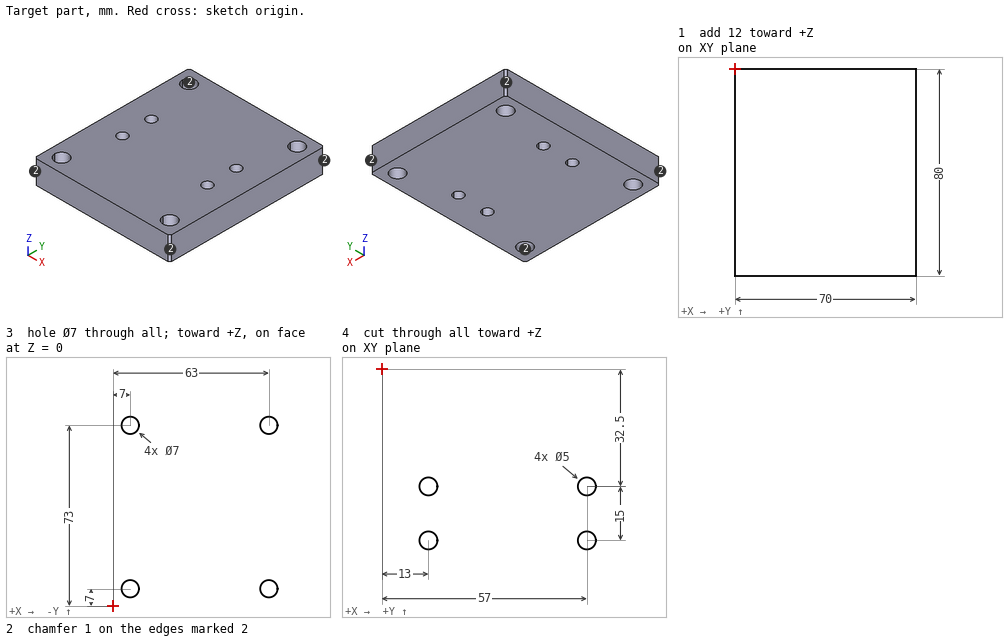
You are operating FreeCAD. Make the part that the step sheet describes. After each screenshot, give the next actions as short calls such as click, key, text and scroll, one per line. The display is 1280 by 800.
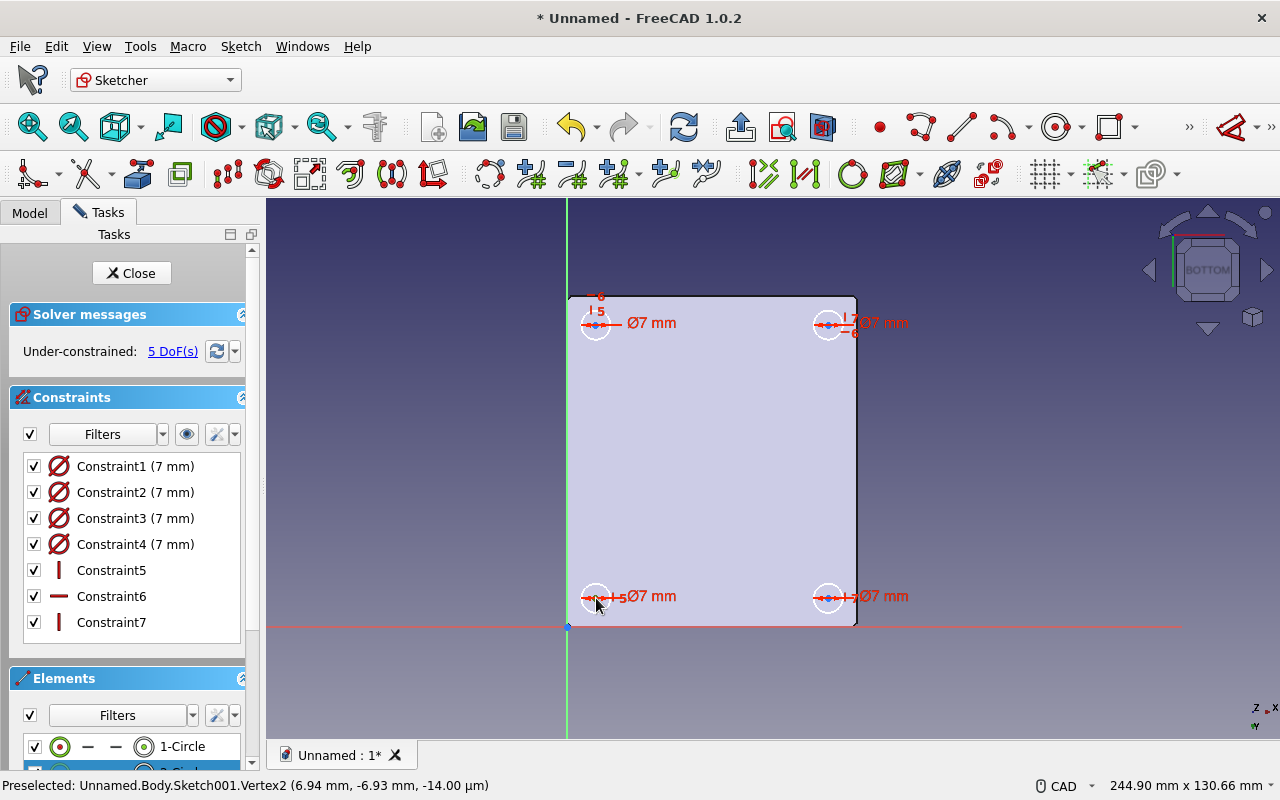
click(828, 598)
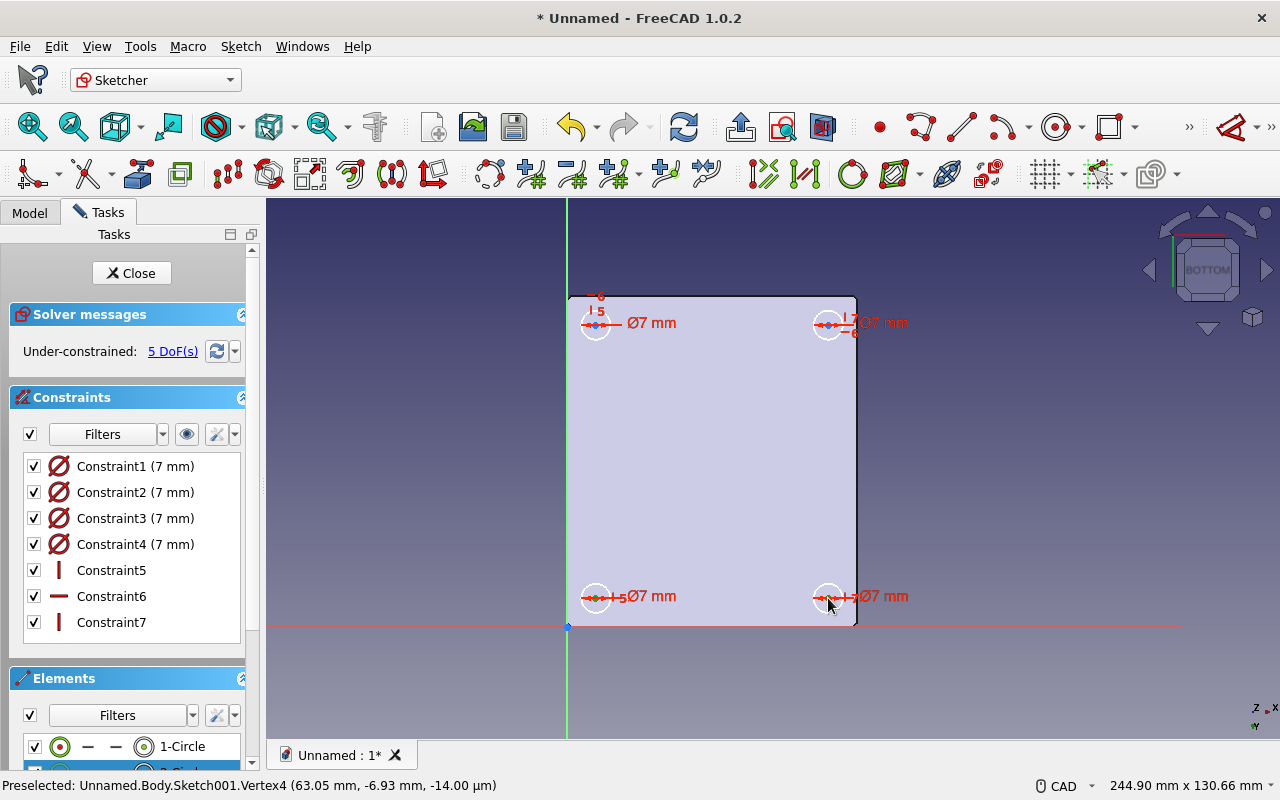
key(h)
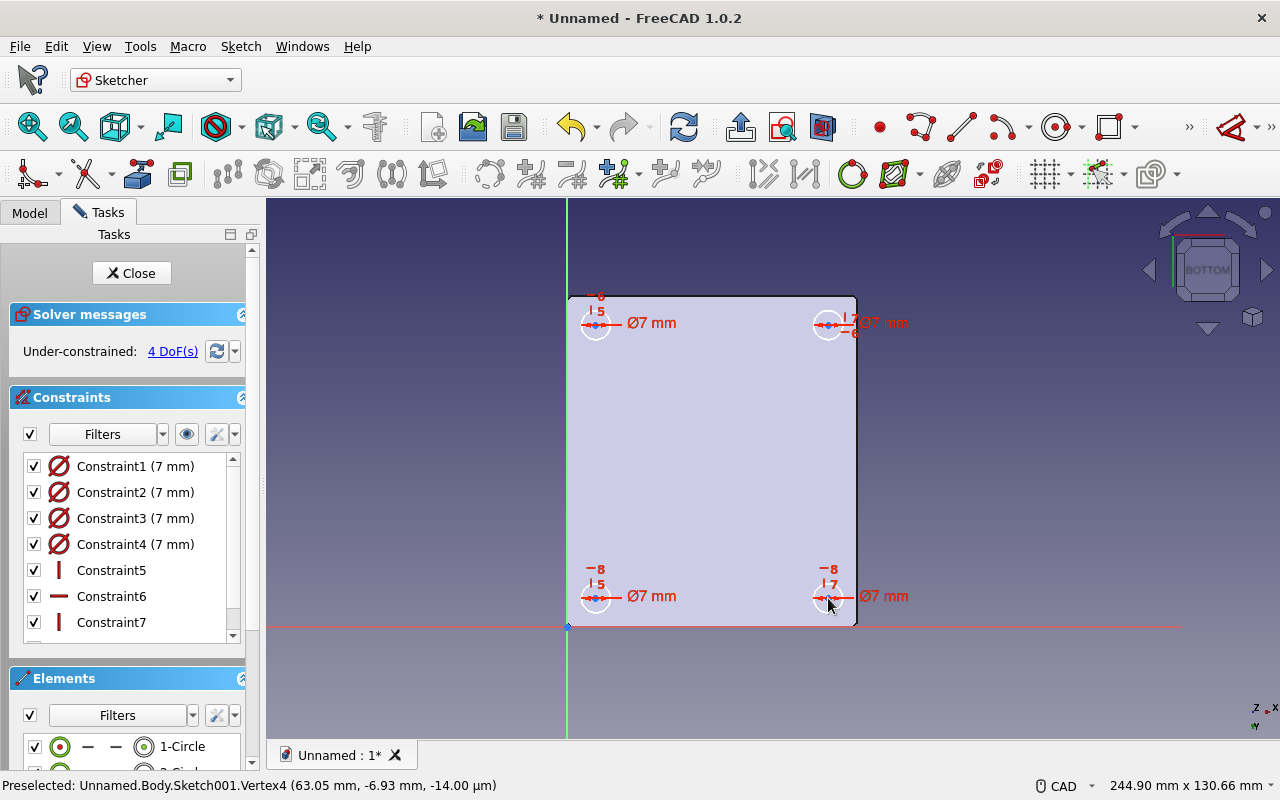
click(1230, 128)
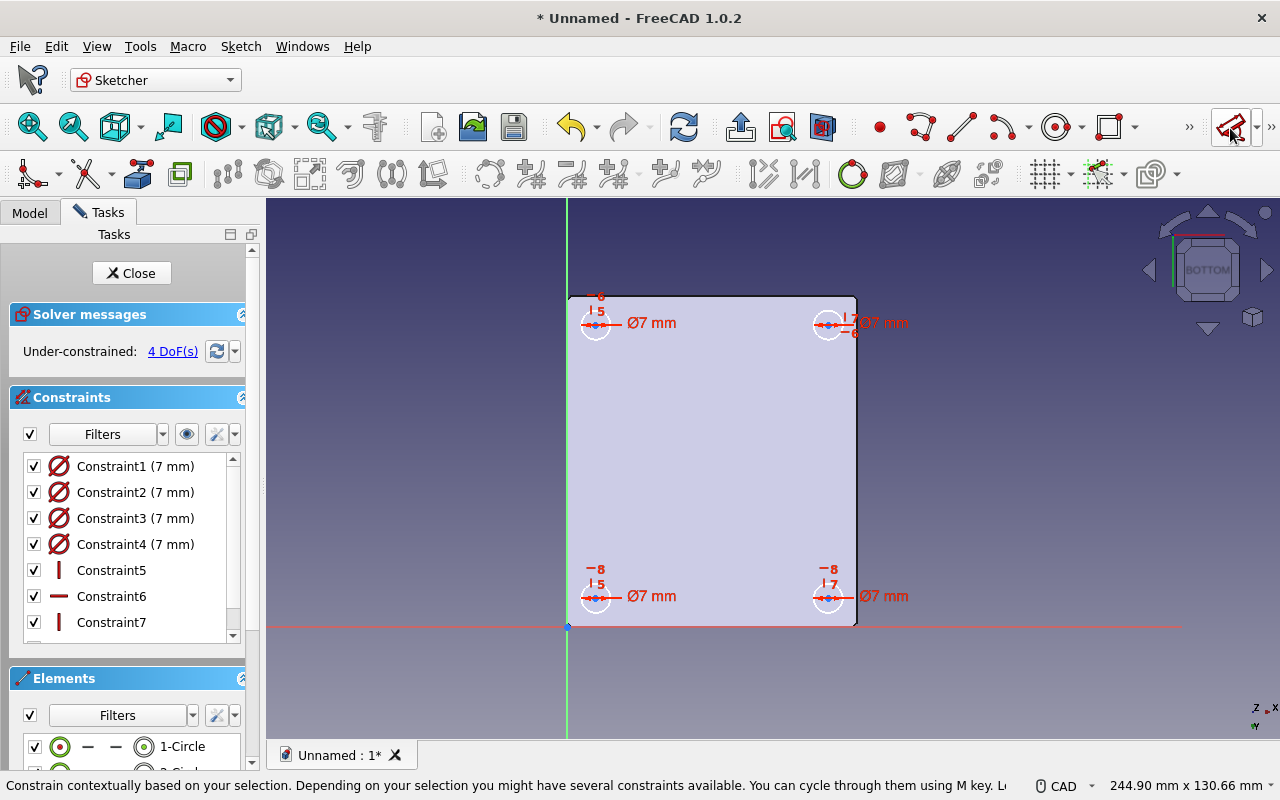
scroll(596, 325, up, 2)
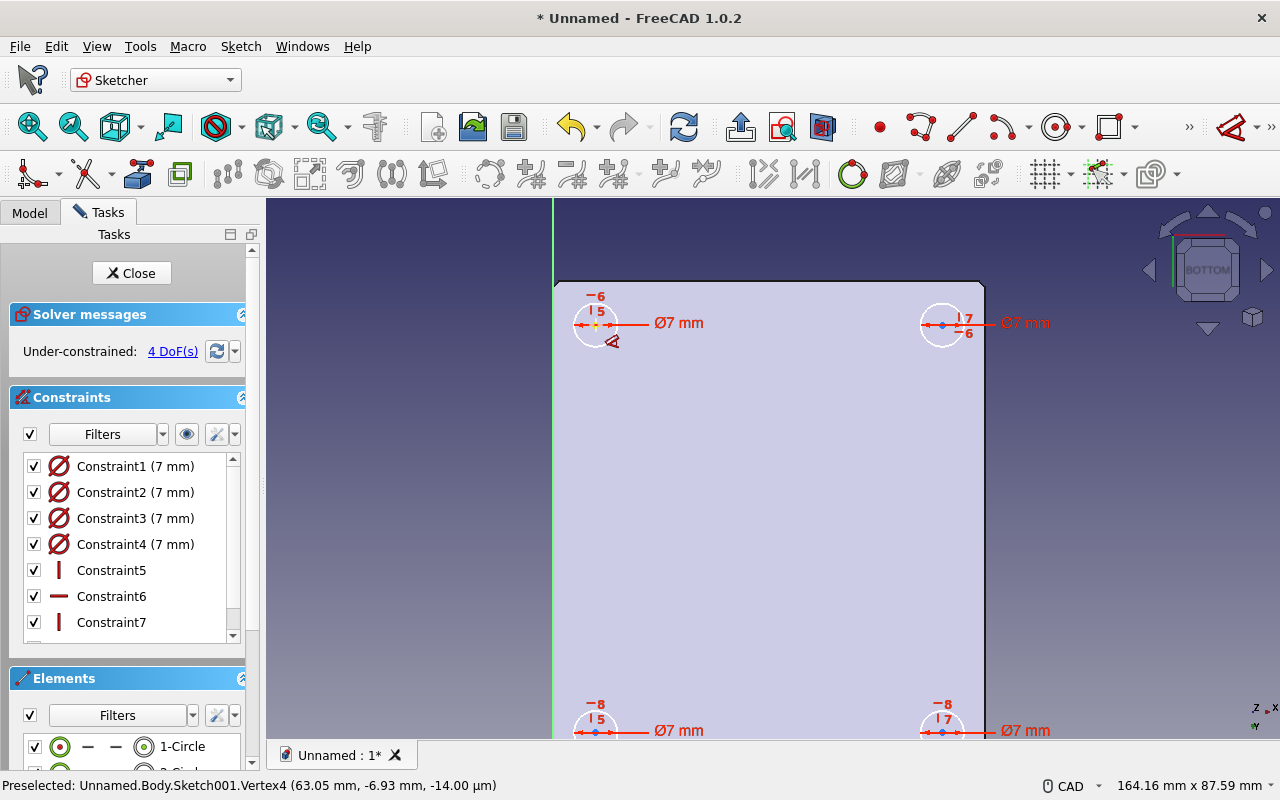
click(596, 325)
click(574, 291)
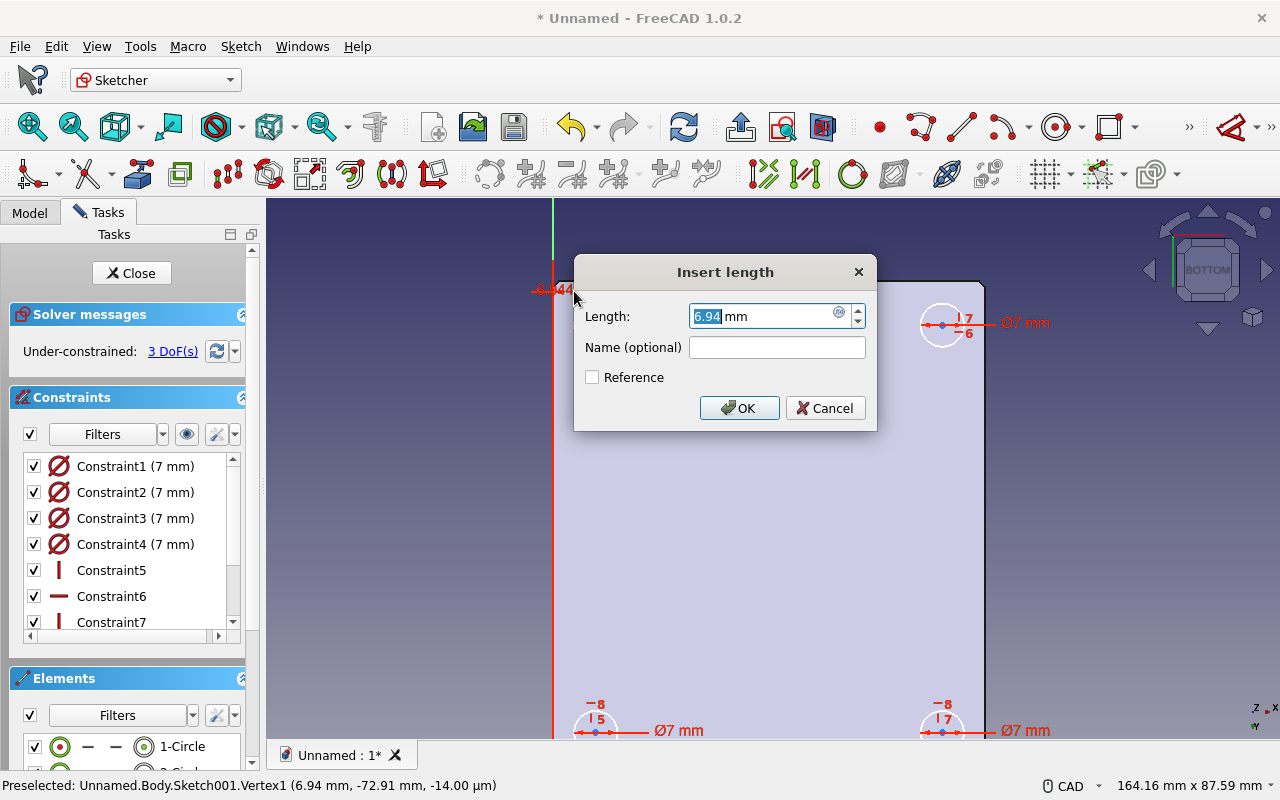
text(7)
key(Return)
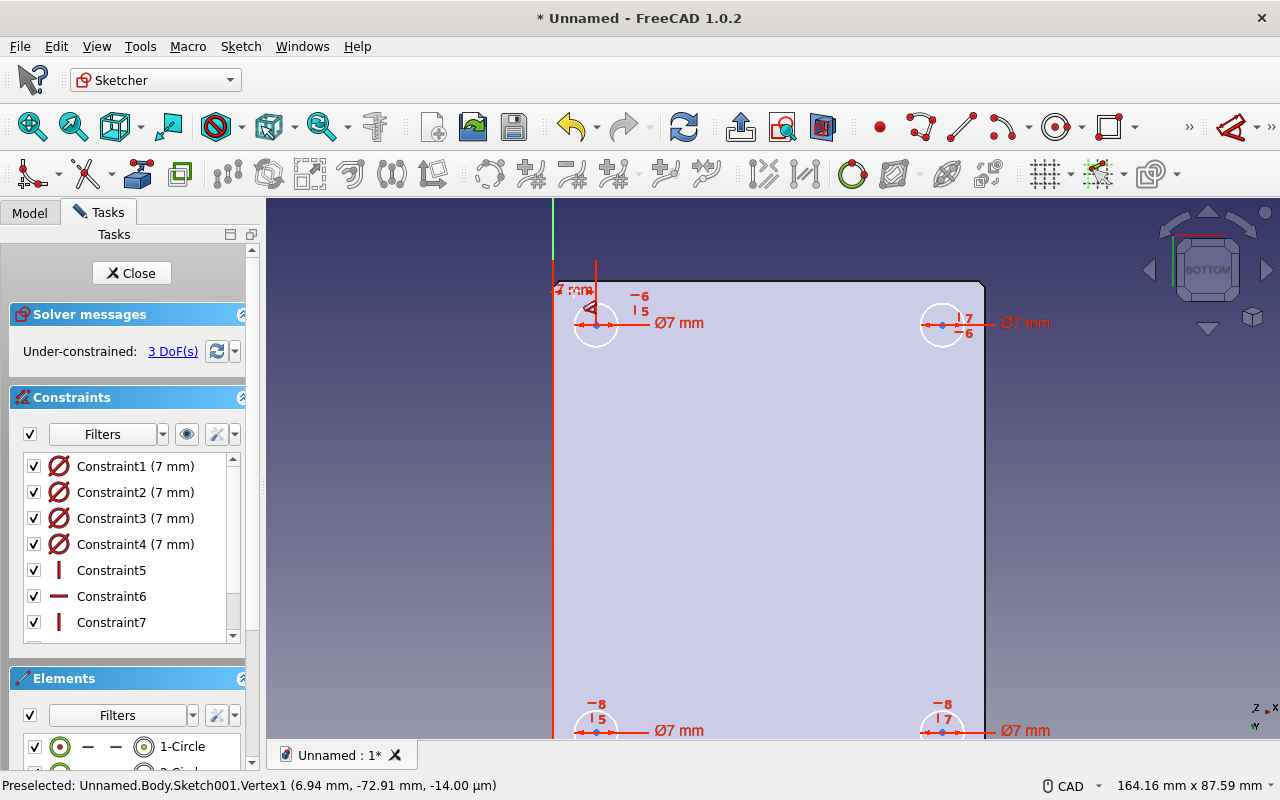
scroll(595, 325, down, 2)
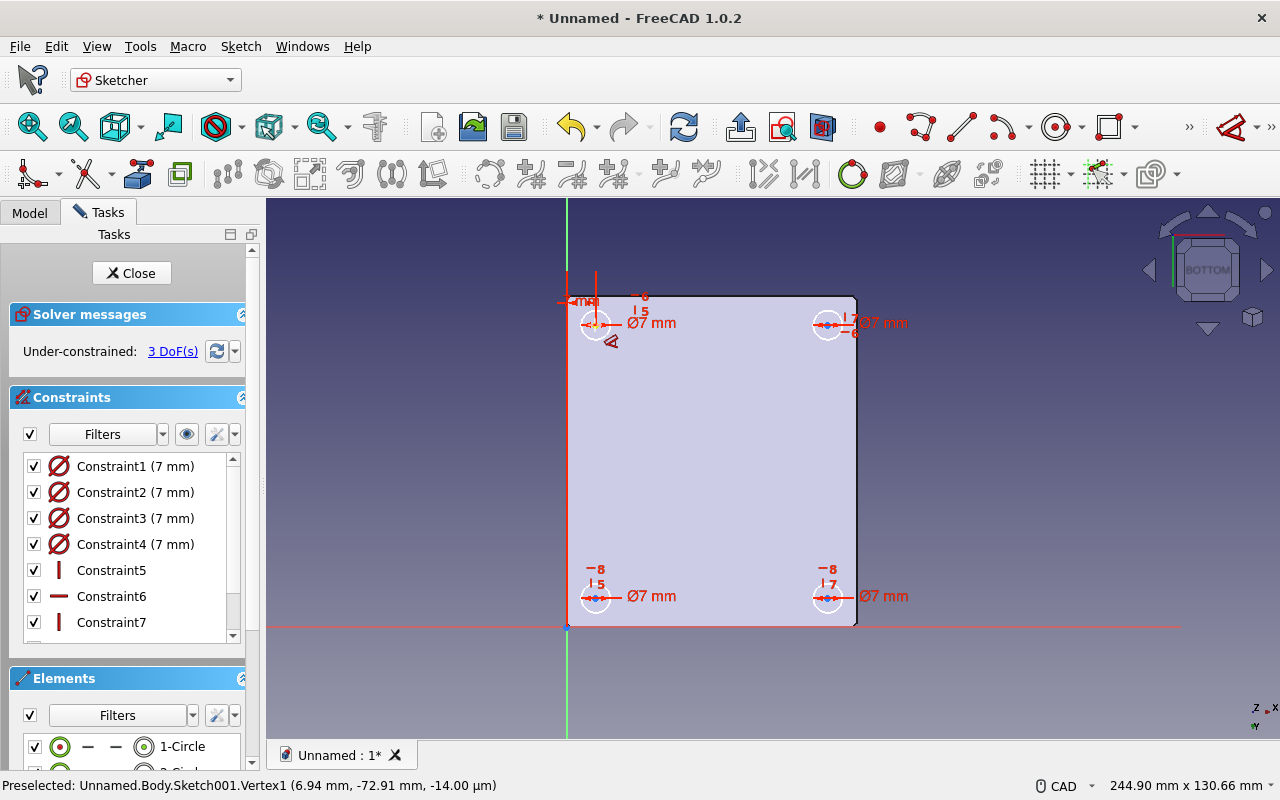
scroll(596, 598, up, 2)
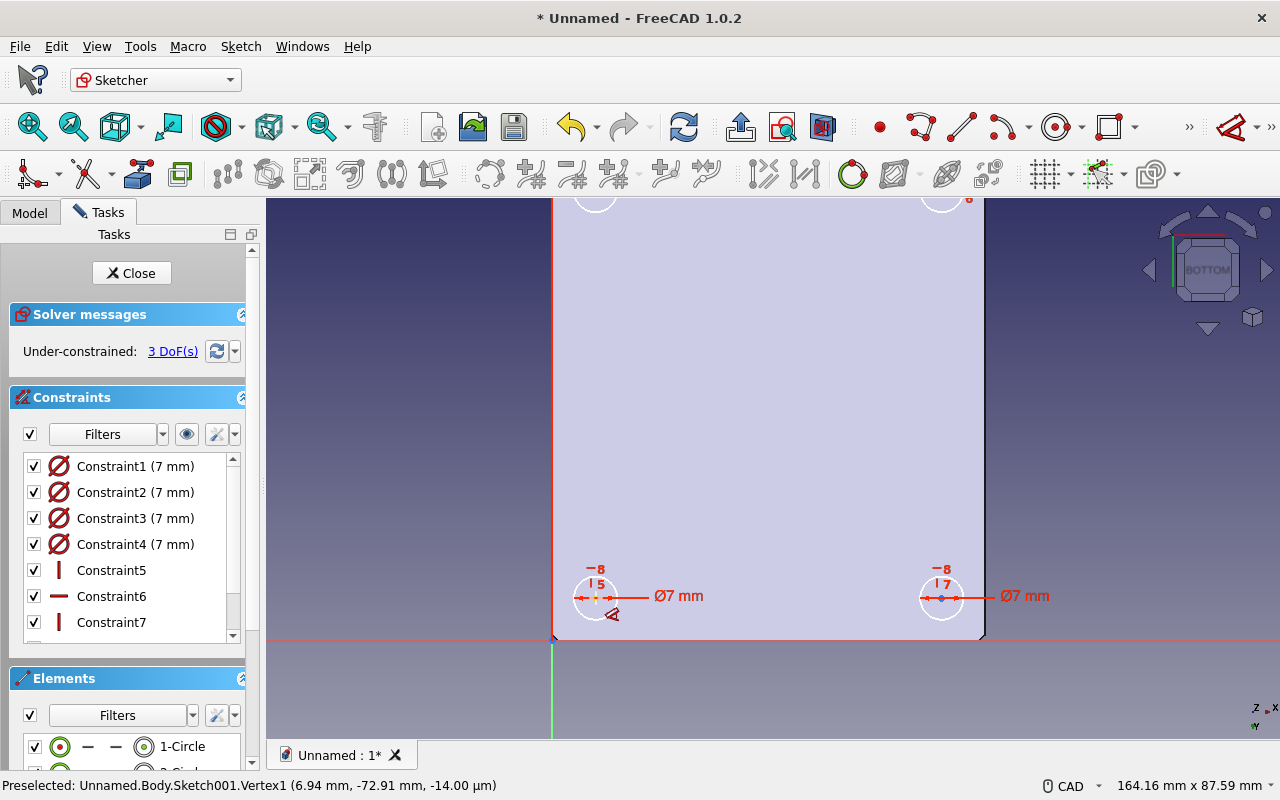
click(596, 598)
click(518, 620)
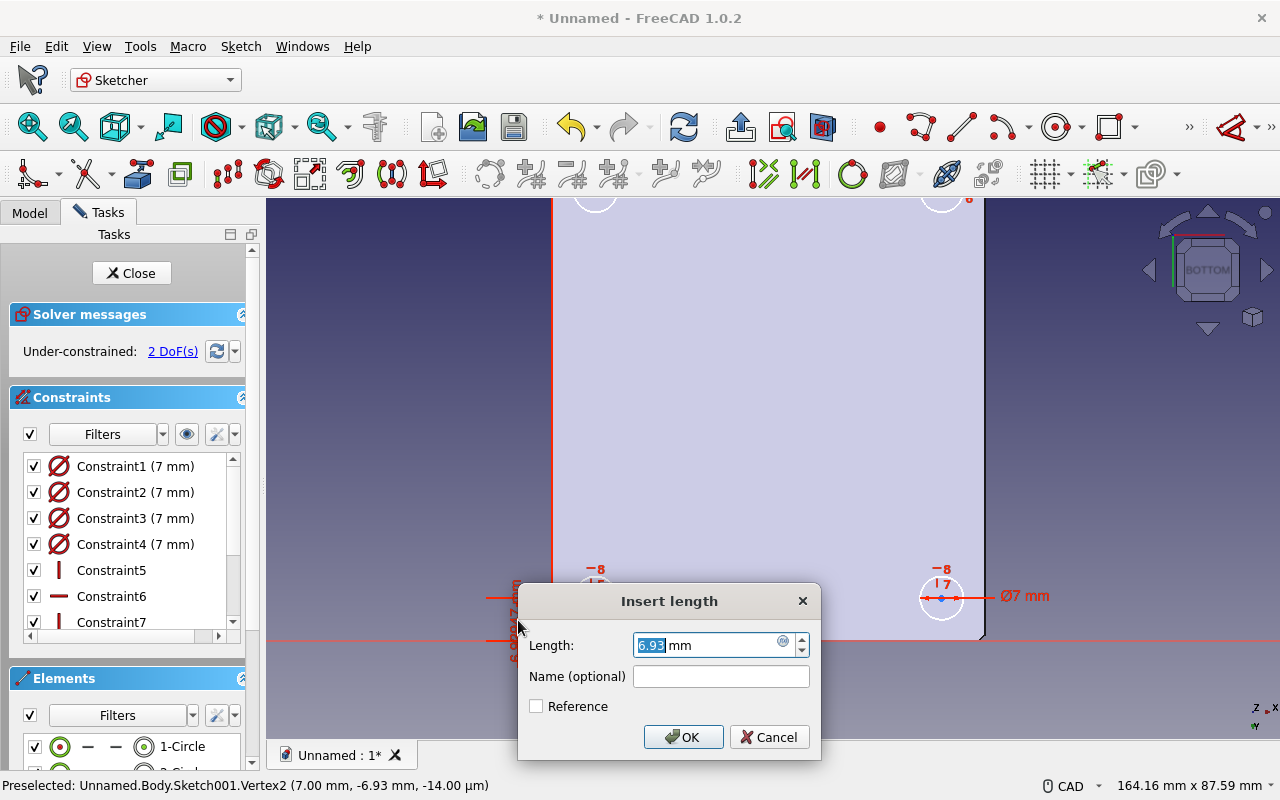
text(7)
key(Return)